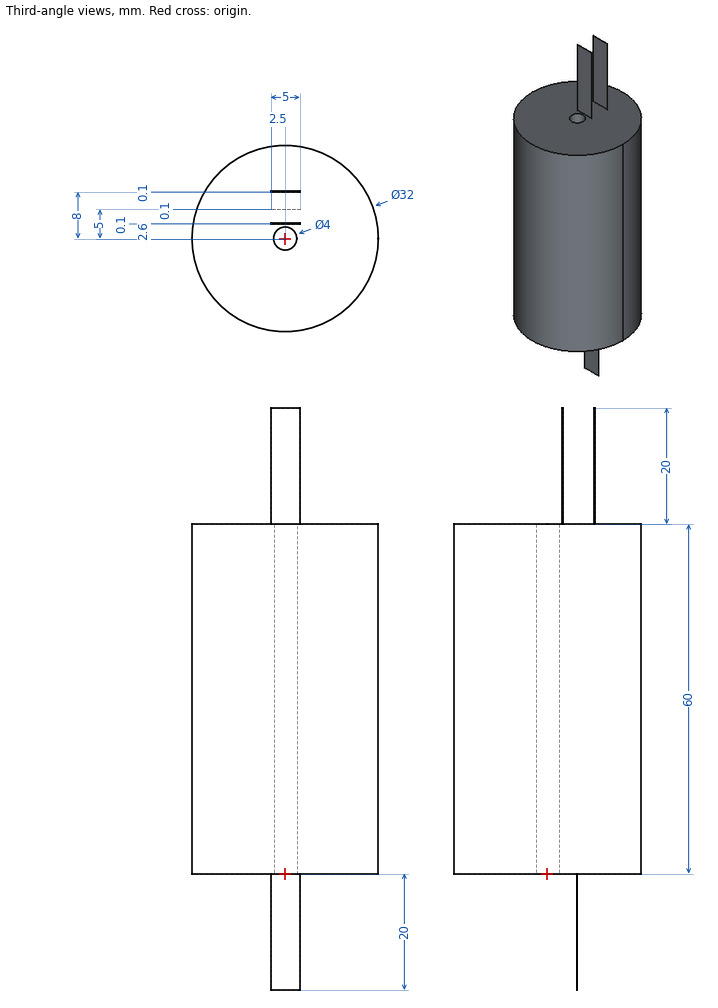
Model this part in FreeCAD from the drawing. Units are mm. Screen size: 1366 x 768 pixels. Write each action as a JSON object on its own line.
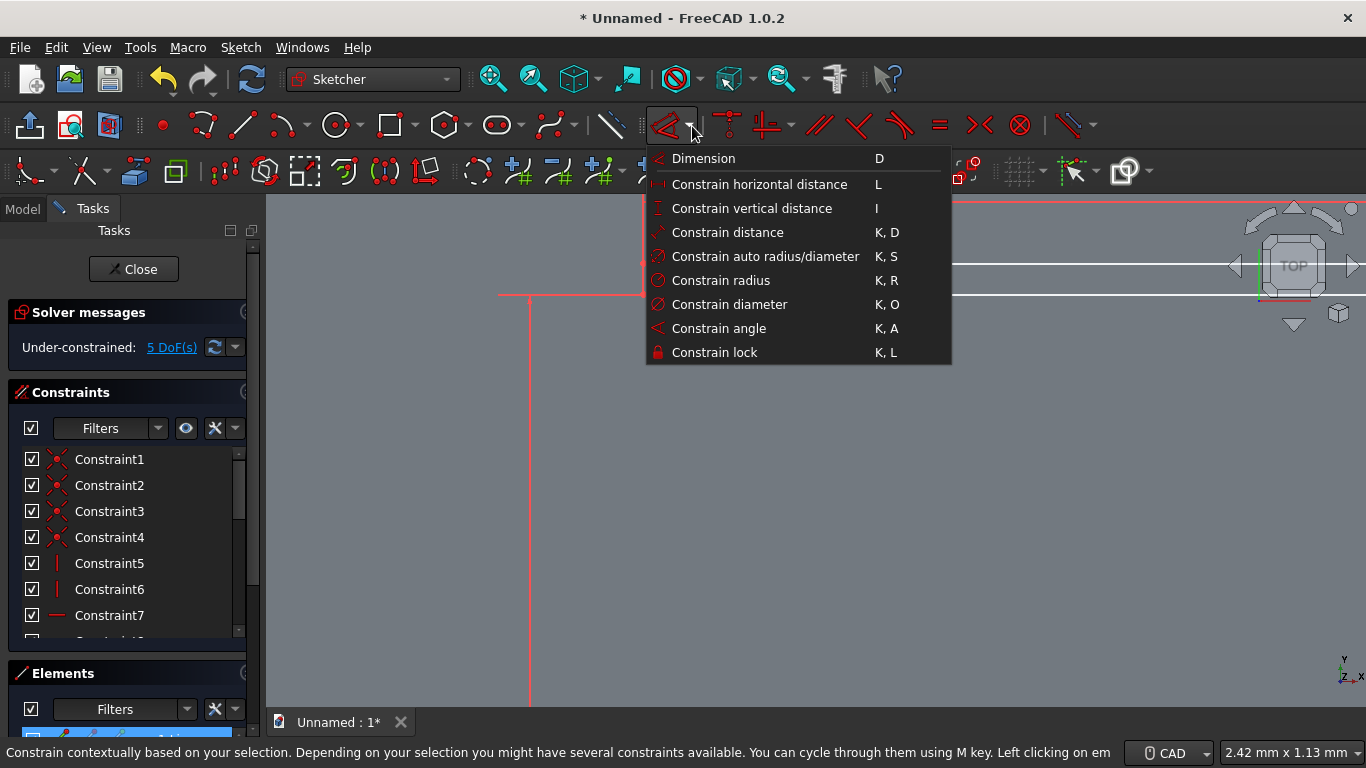
{"action": "left_click", "coordinate": [799, 208]}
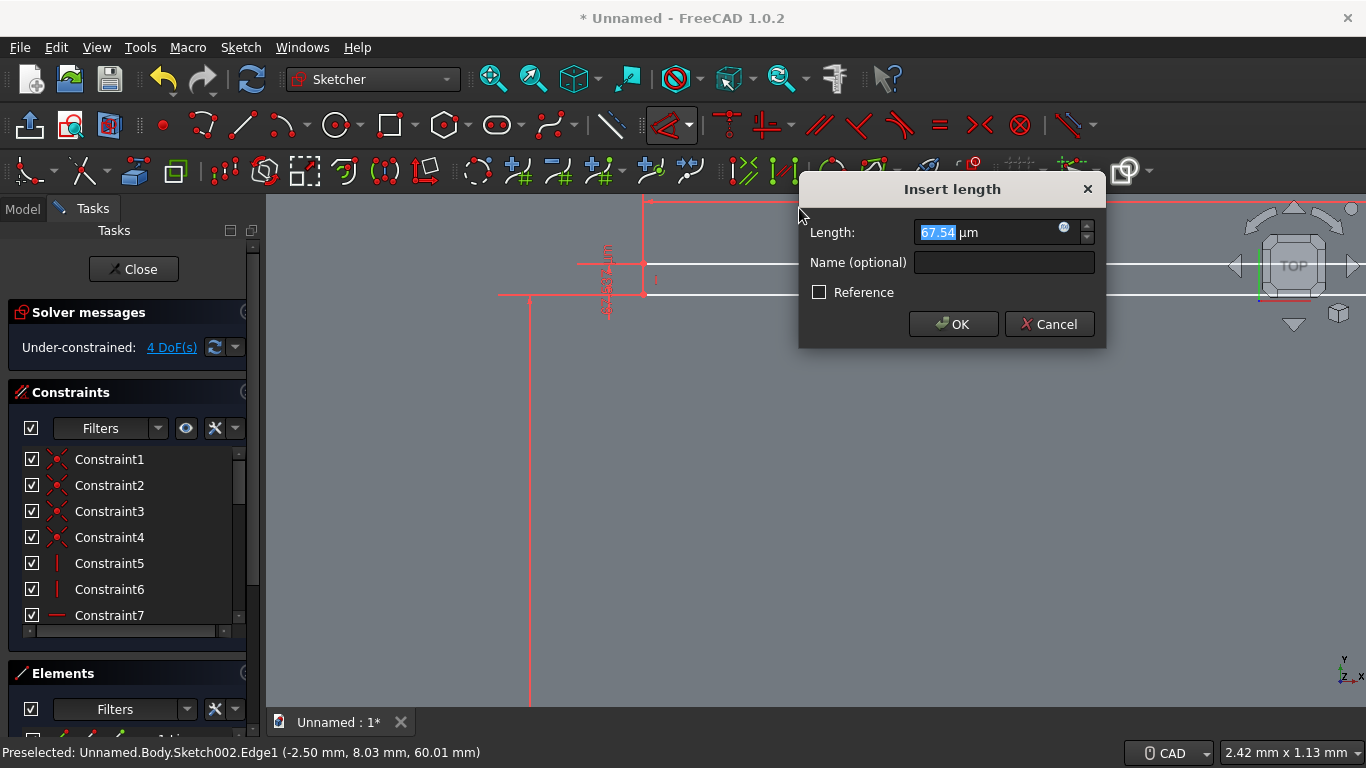
{"action": "key", "text": "ctrl+a"}
{"action": "type", "text": "0.1 mm"}
{"action": "key", "text": "Return"}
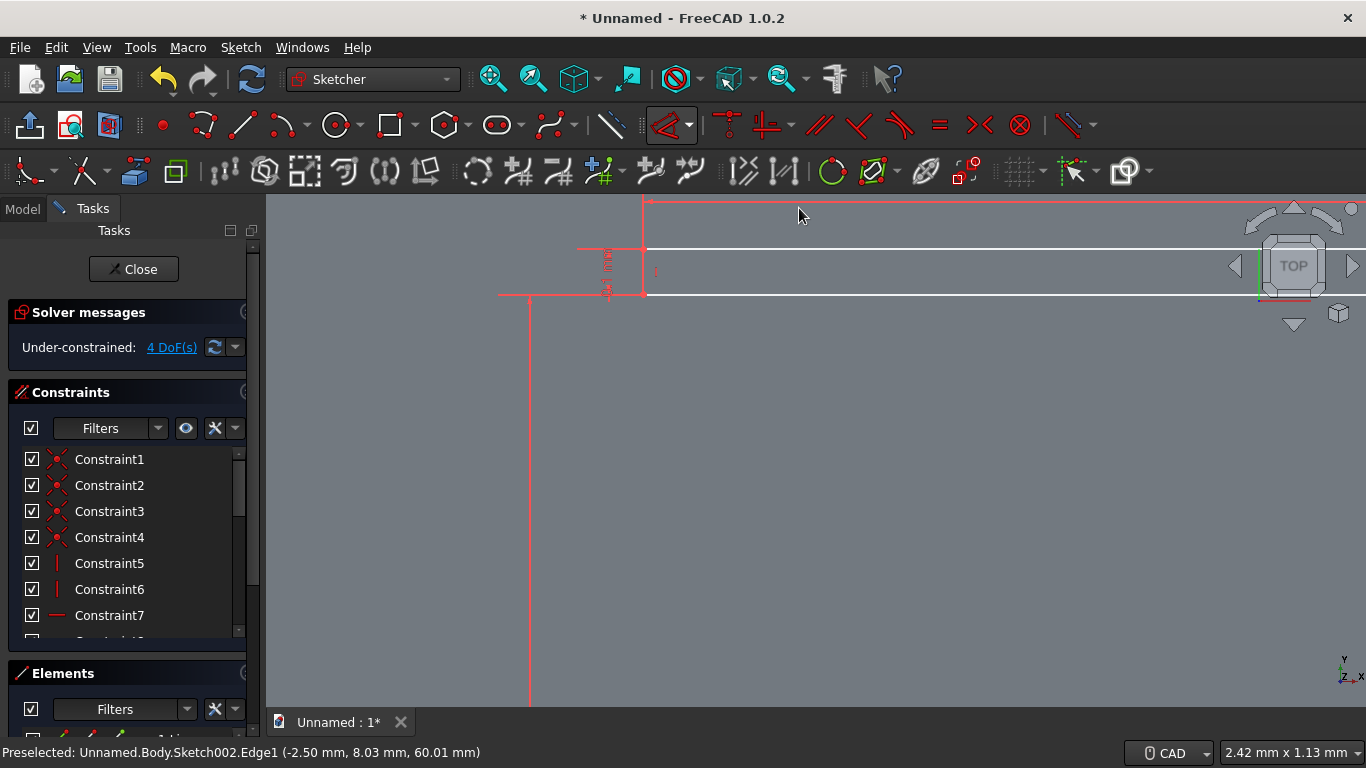
{"action": "scroll", "coordinate": [645, 287], "scroll_direction": "down", "scroll_amount": 12}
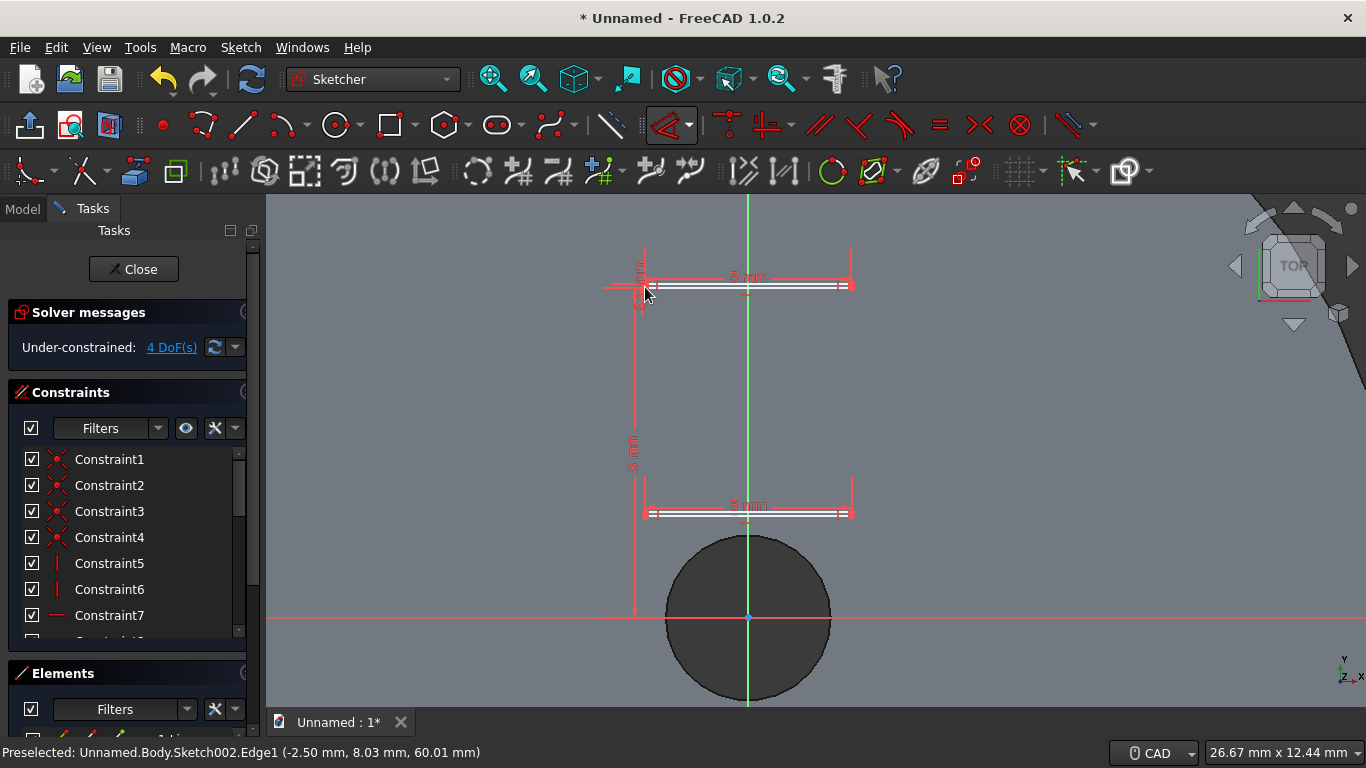
{"action": "scroll", "coordinate": [645, 513], "scroll_direction": "up", "scroll_amount": 13}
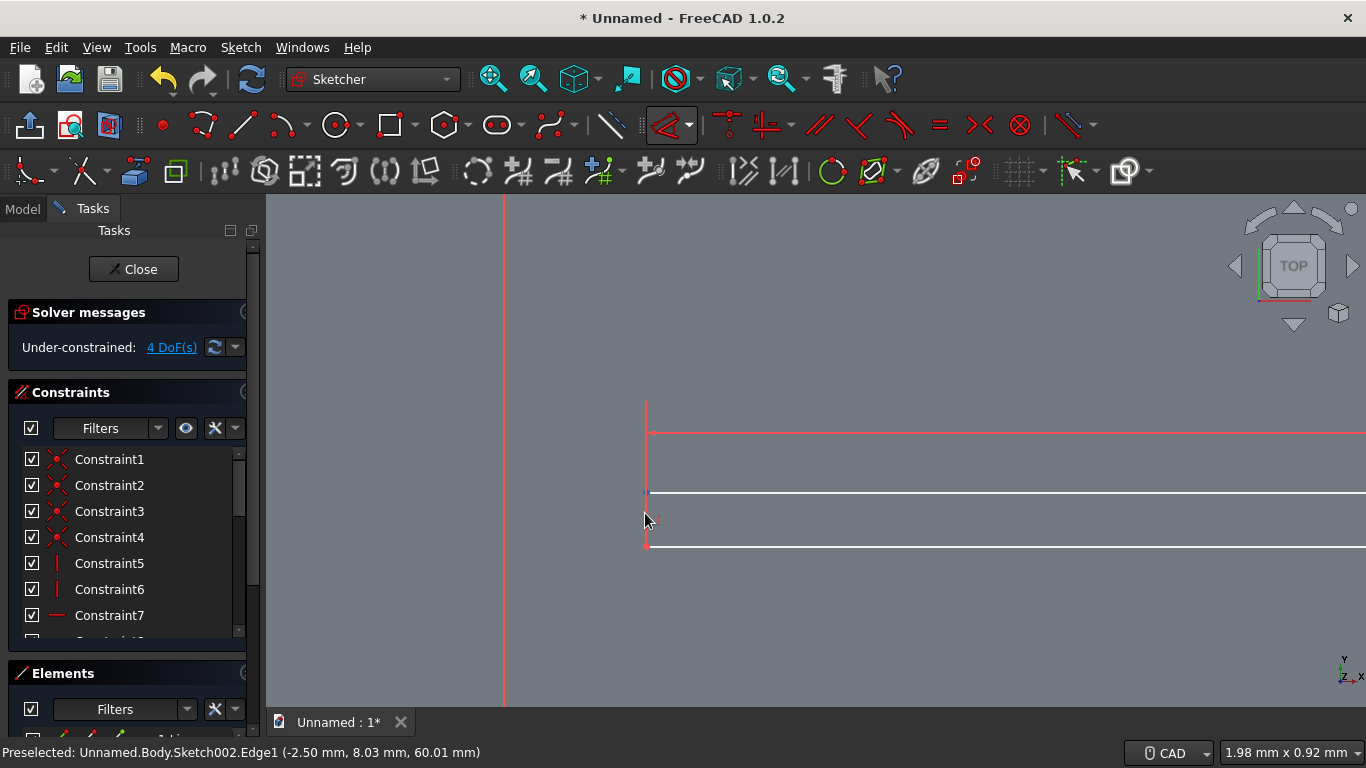
{"action": "left_click", "coordinate": [646, 509]}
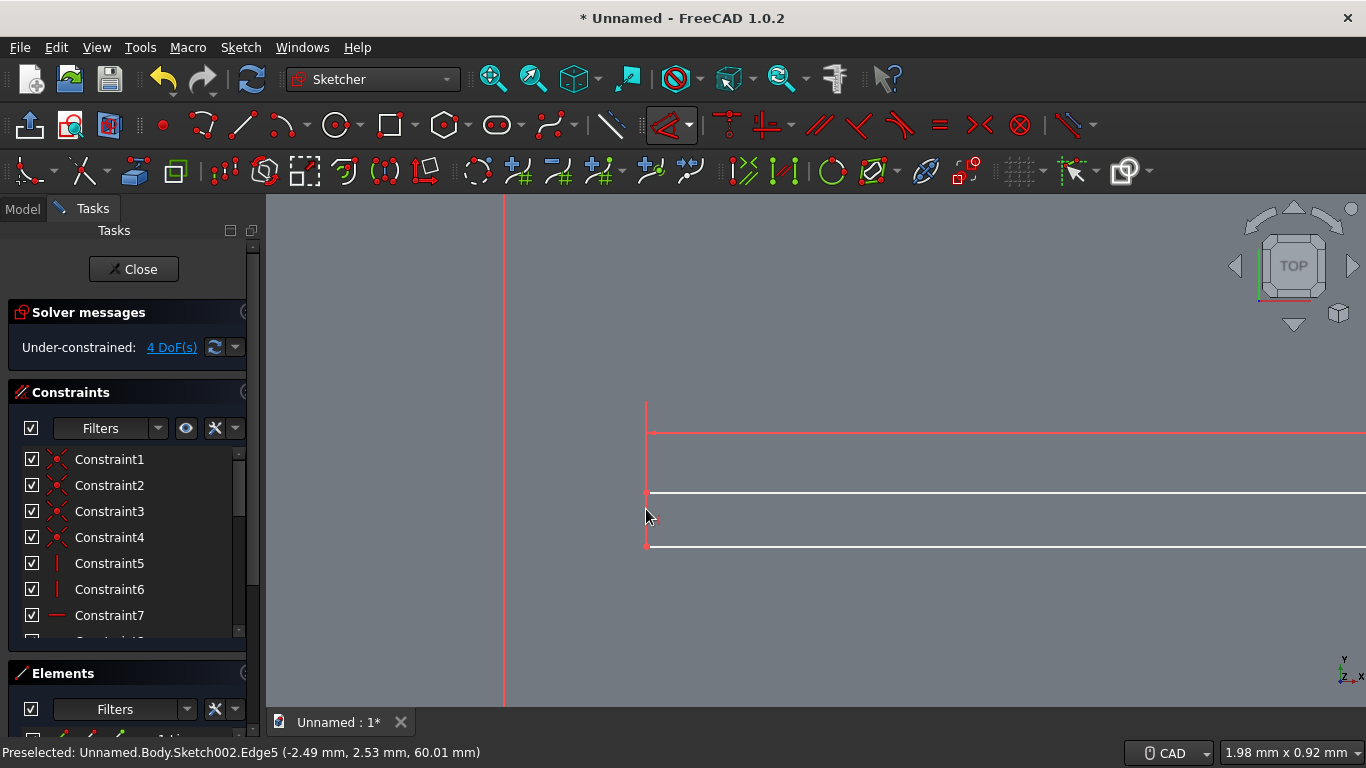
{"action": "left_click", "coordinate": [692, 126]}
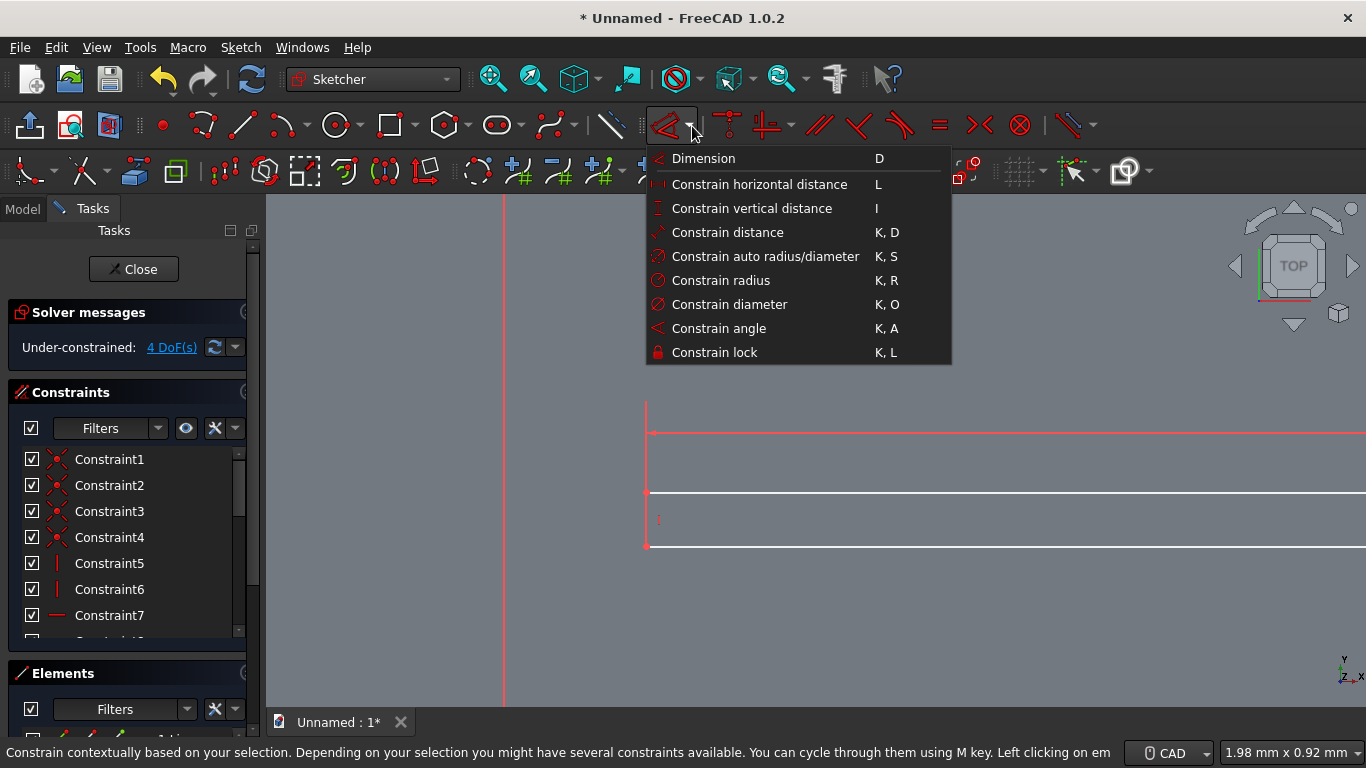
{"action": "left_click", "coordinate": [799, 208]}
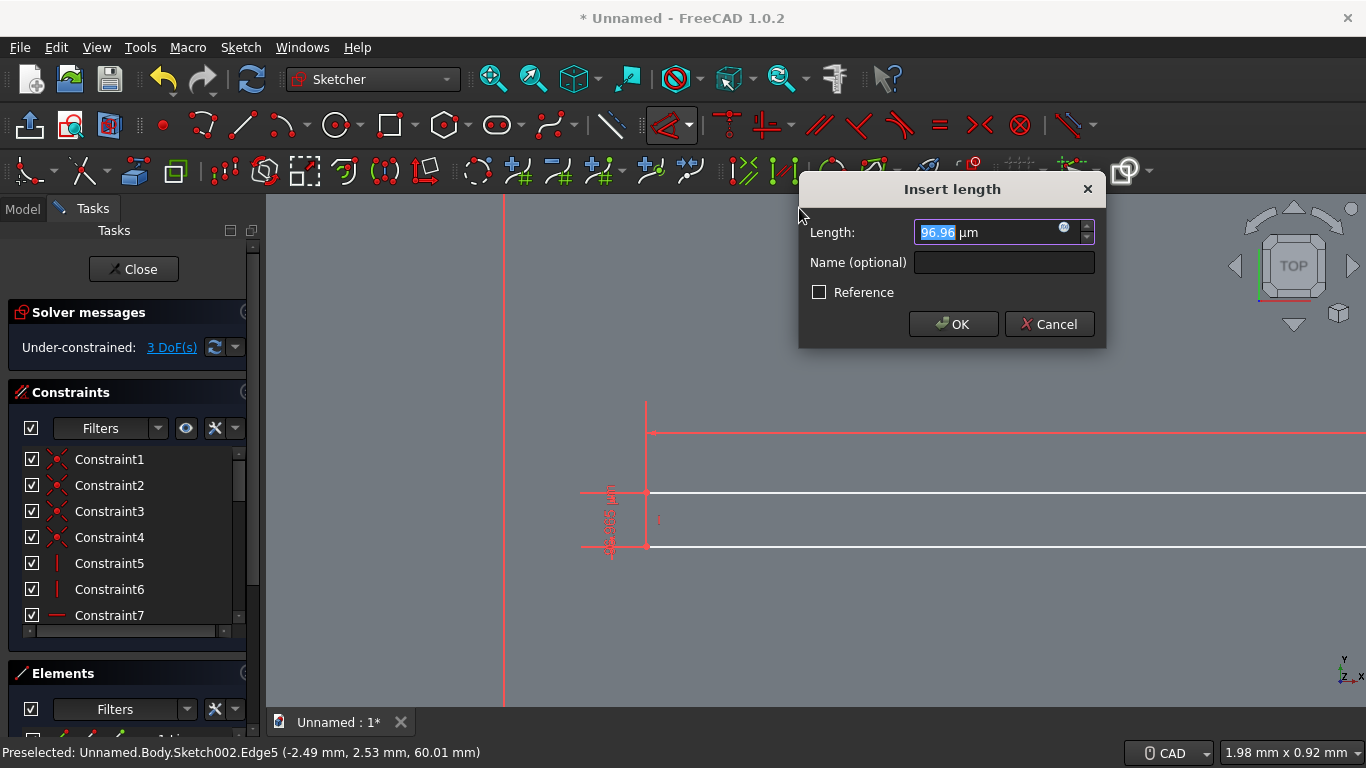
{"action": "key", "text": "ctrl+a"}
{"action": "type", "text": "0.1 mm"}
{"action": "key", "text": "Return"}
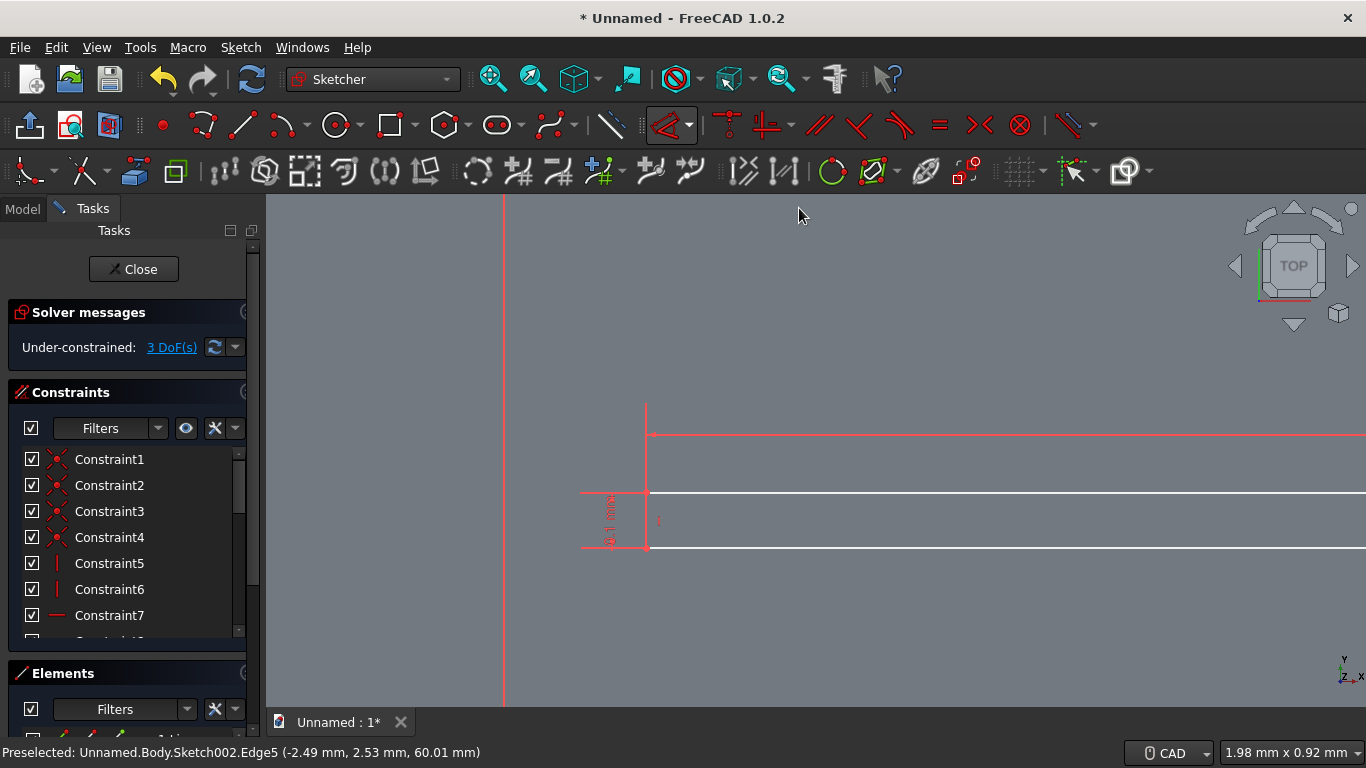
{"action": "scroll", "coordinate": [645, 513], "scroll_direction": "down", "scroll_amount": 13}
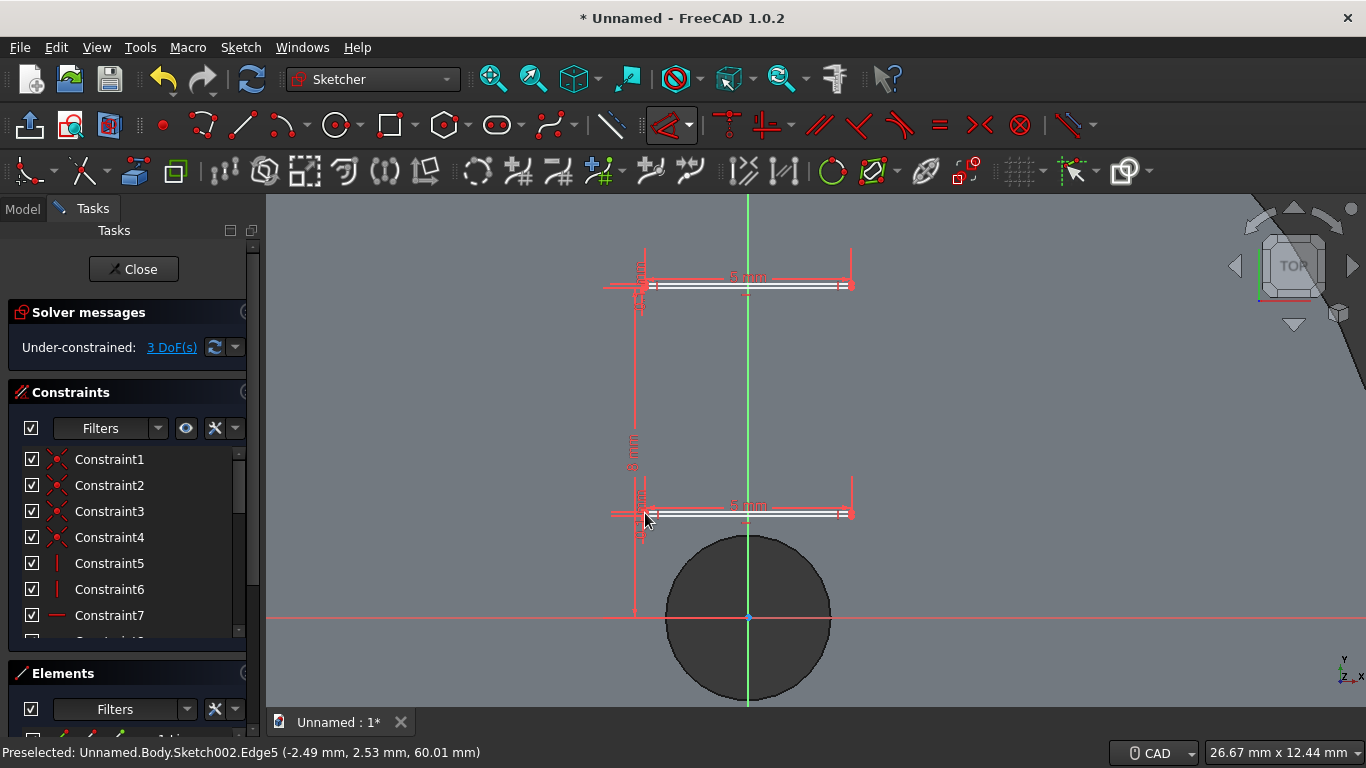
{"action": "scroll", "coordinate": [645, 284], "scroll_direction": "up", "scroll_amount": 6}